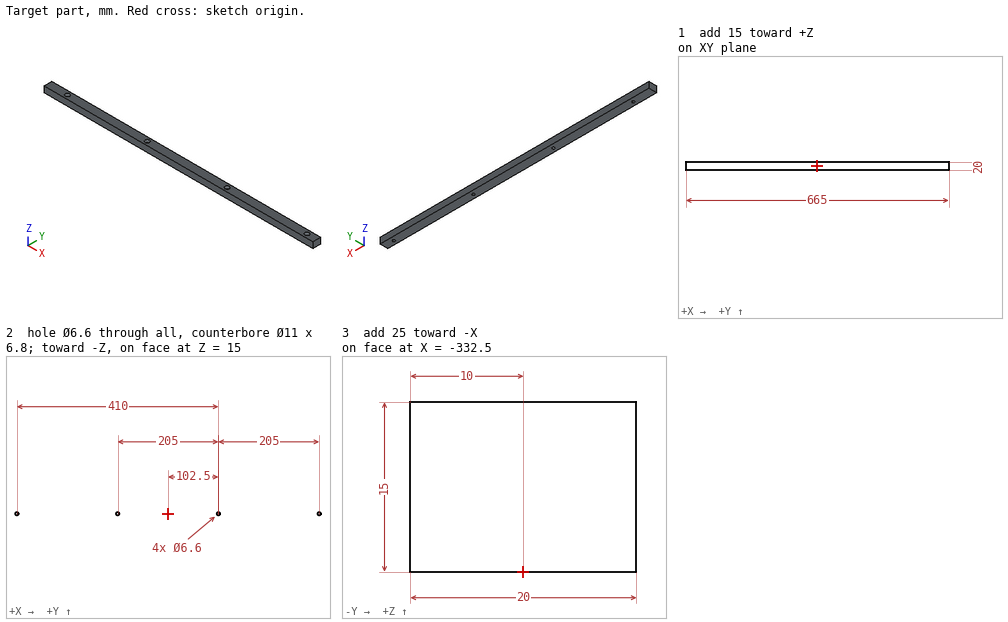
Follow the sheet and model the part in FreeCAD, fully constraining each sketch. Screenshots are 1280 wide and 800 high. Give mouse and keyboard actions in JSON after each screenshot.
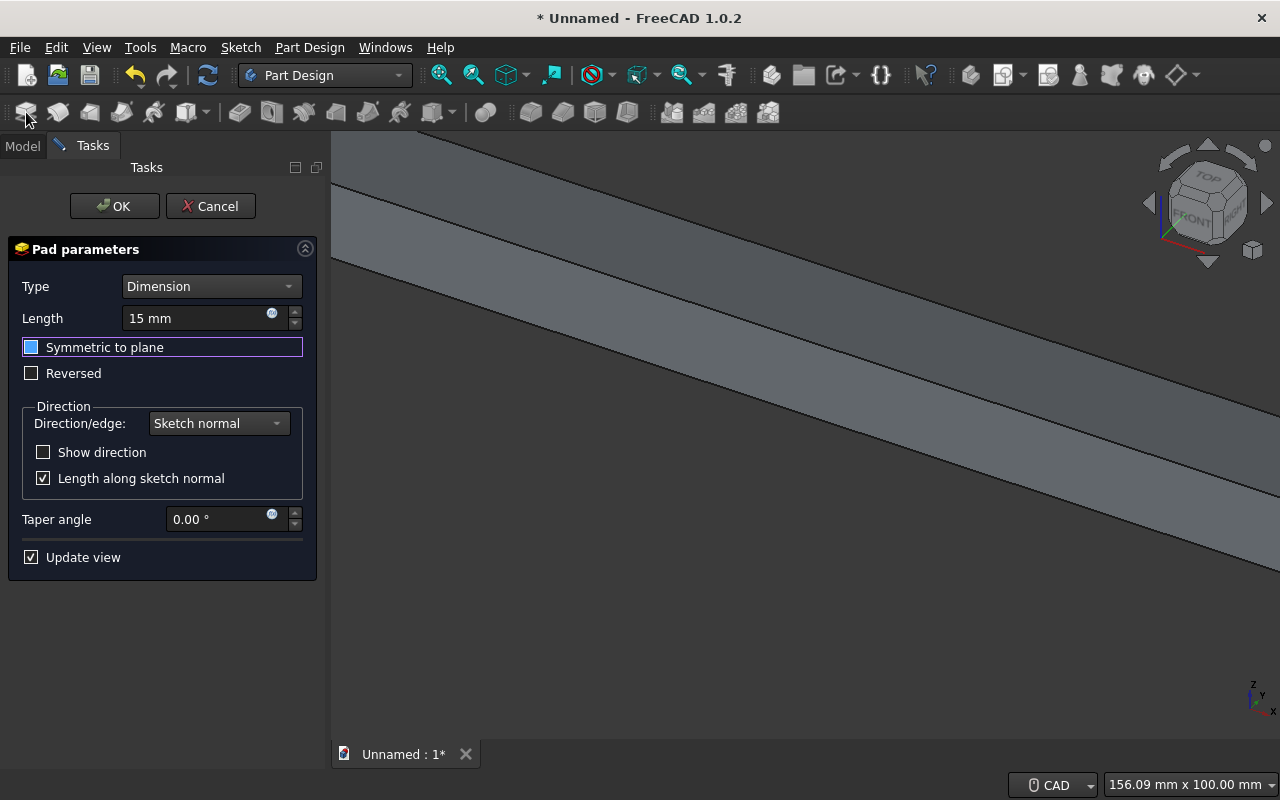
{"action": "left_click", "coordinate": [115, 206]}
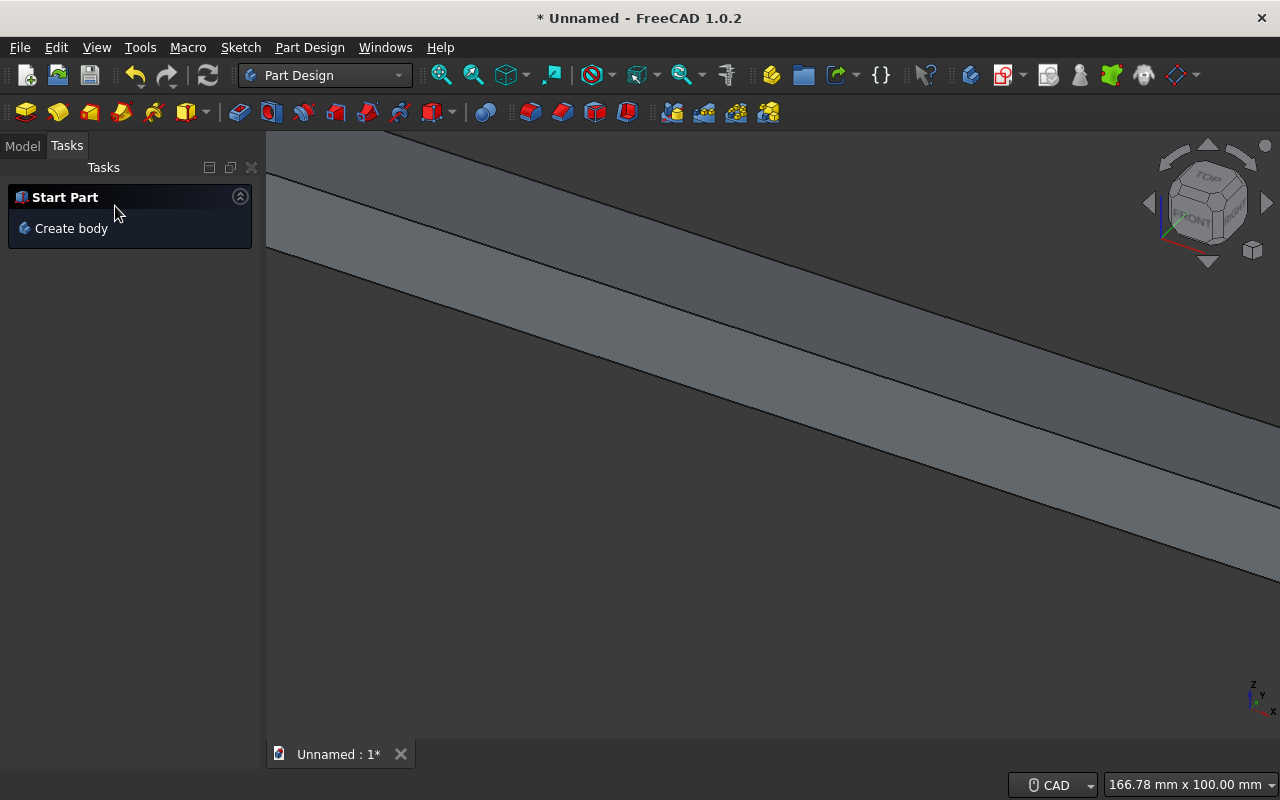
{"action": "key", "text": "v f"}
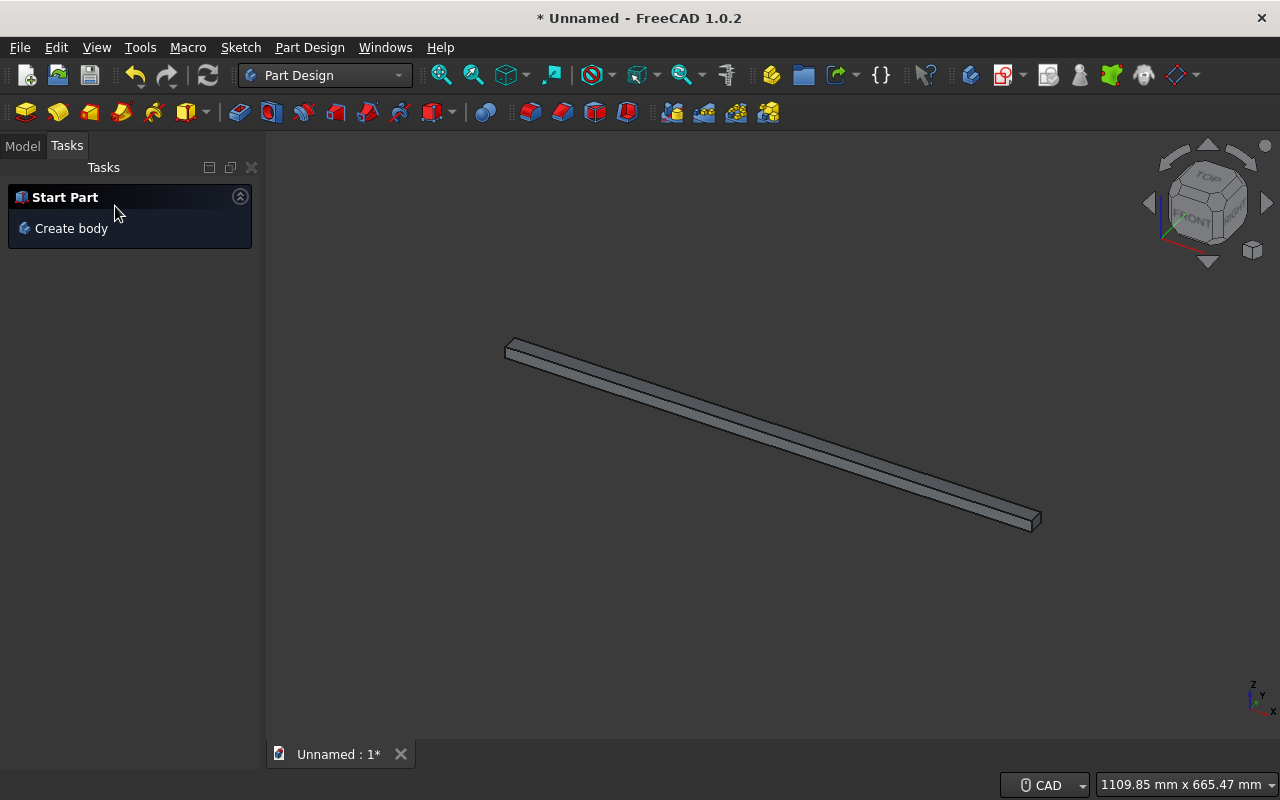
{"action": "key", "text": "0"}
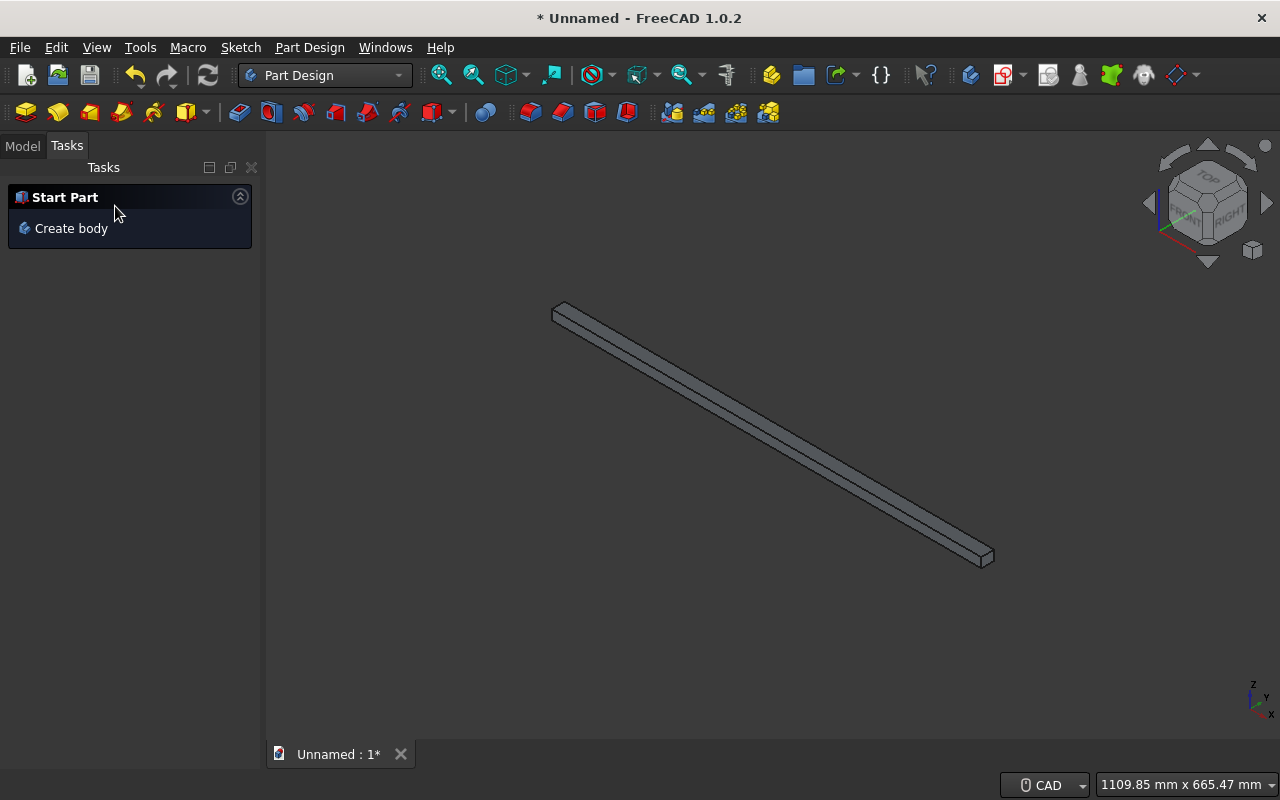
{"action": "key", "text": "v f"}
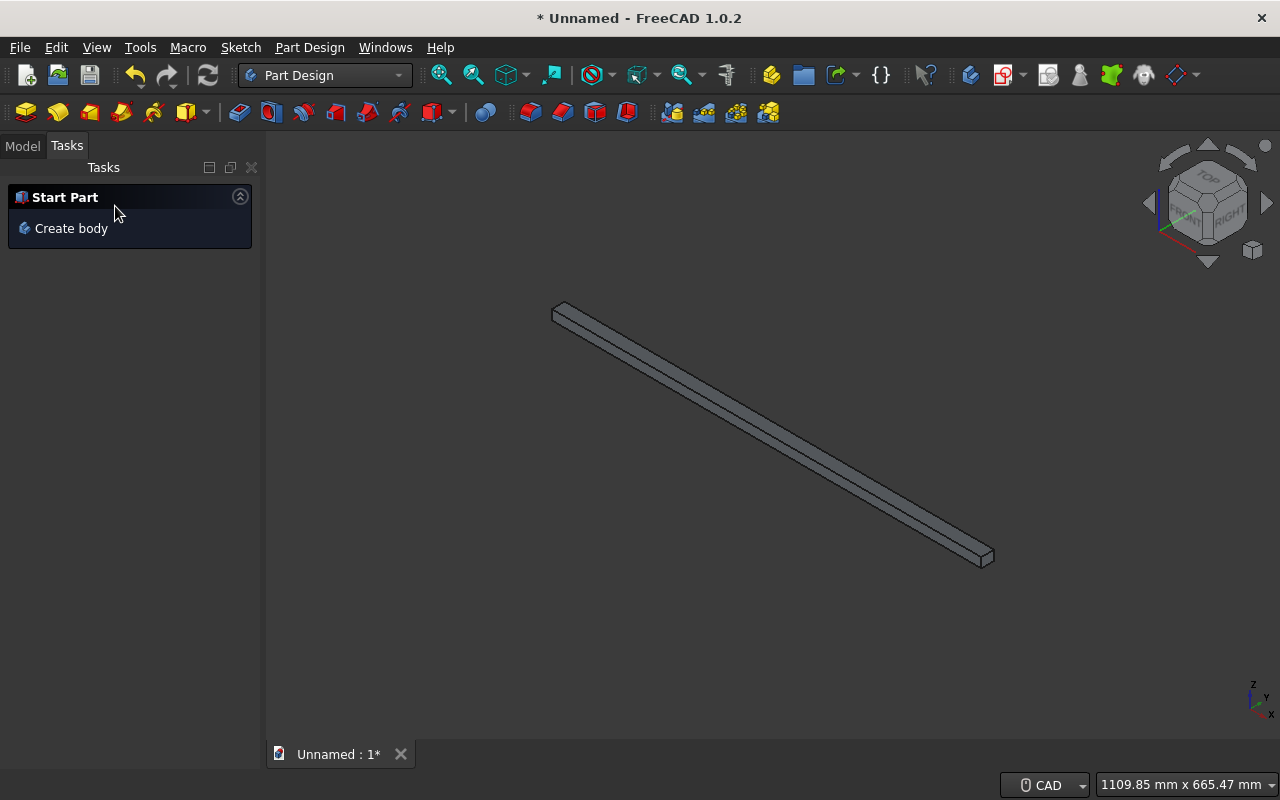
{"action": "key", "text": "2"}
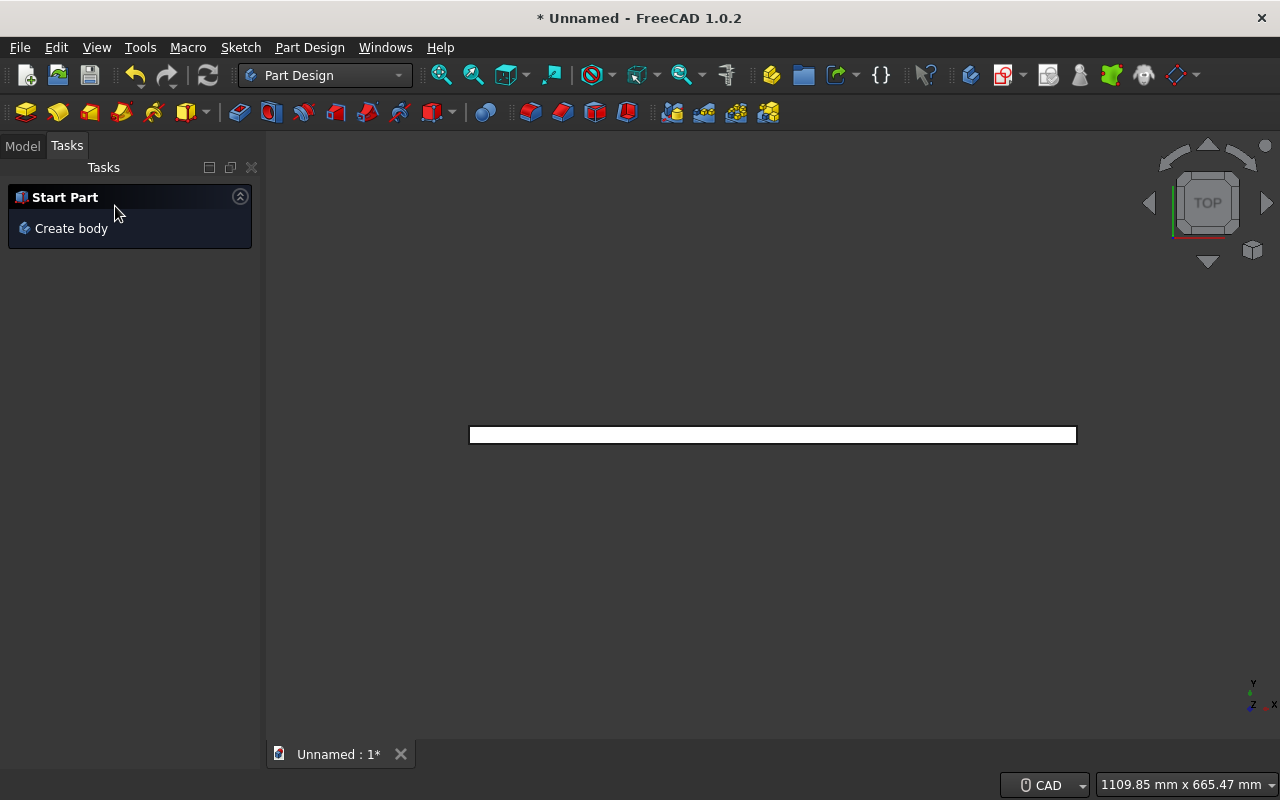
{"action": "left_click", "coordinate": [1033, 434]}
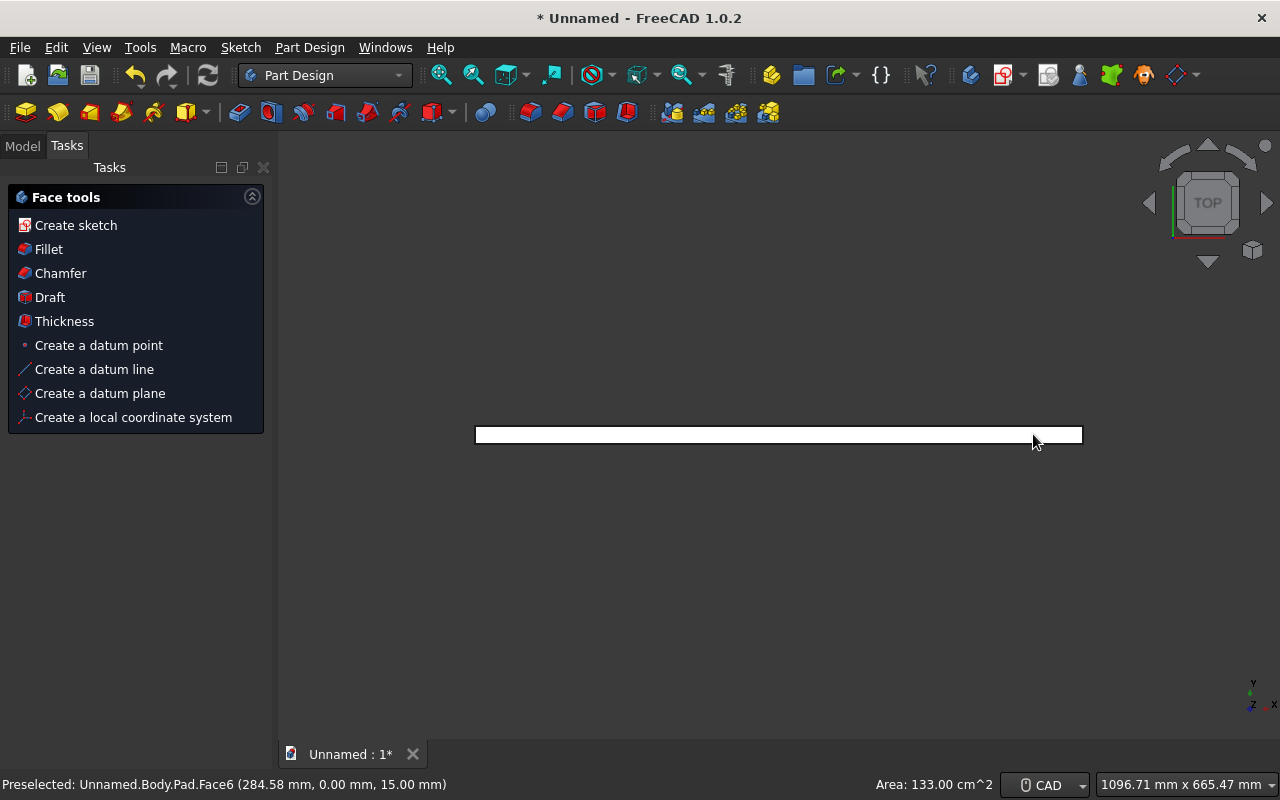
{"action": "left_click", "coordinate": [1004, 76]}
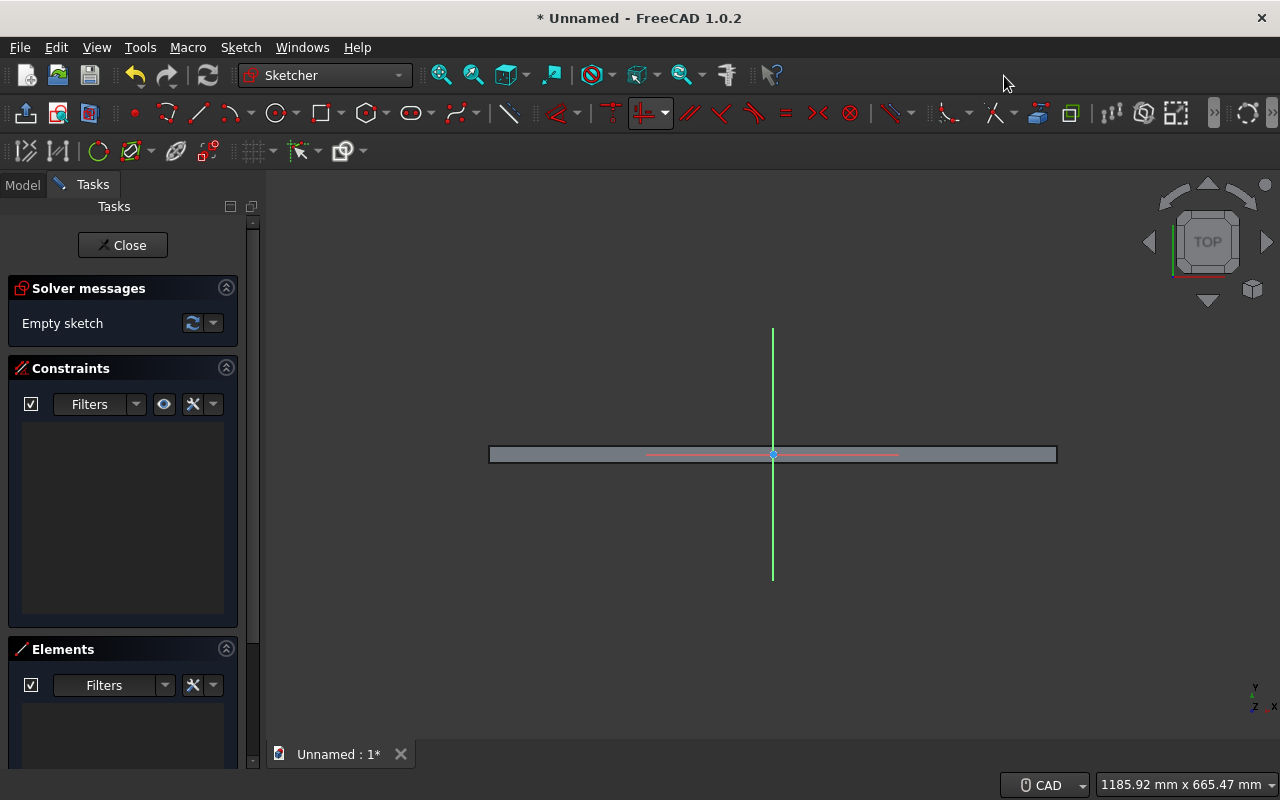
{"action": "left_click", "coordinate": [276, 114]}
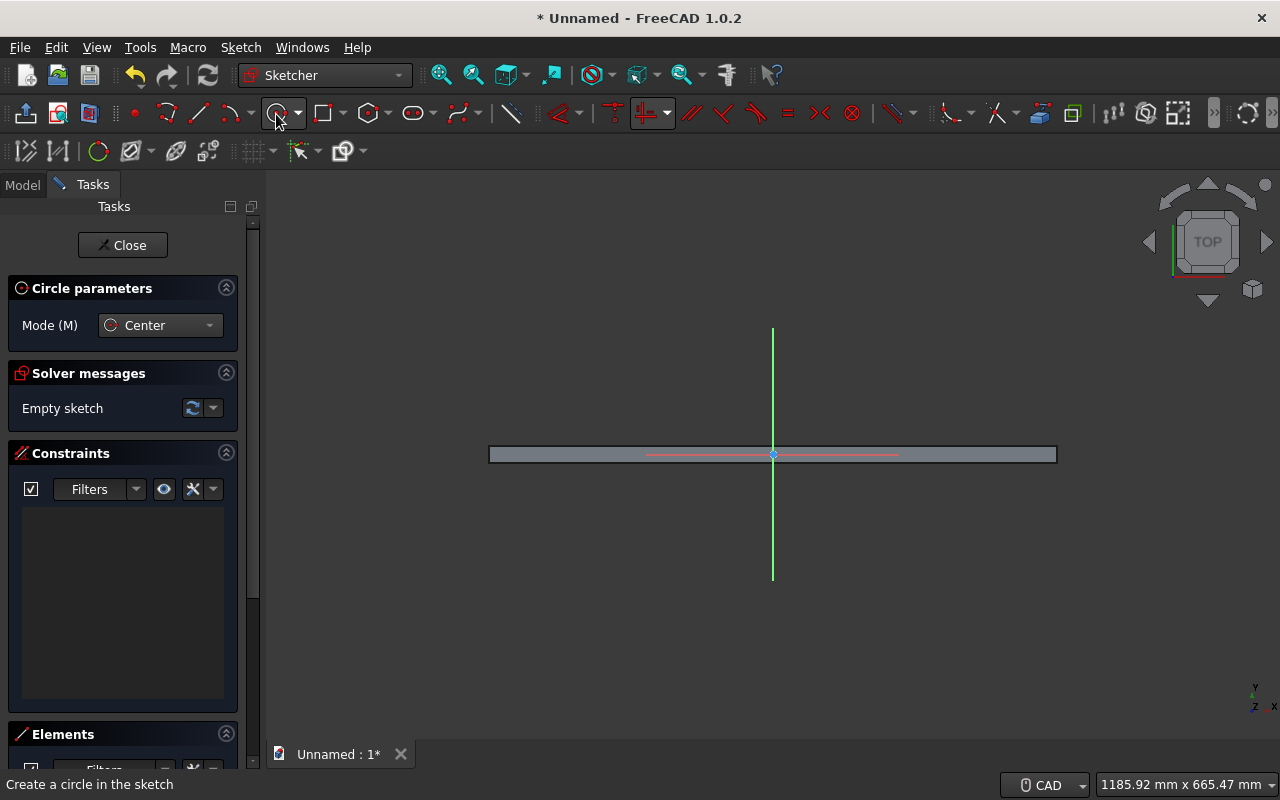
{"action": "scroll", "coordinate": [861, 454], "scroll_direction": "up", "scroll_amount": 11}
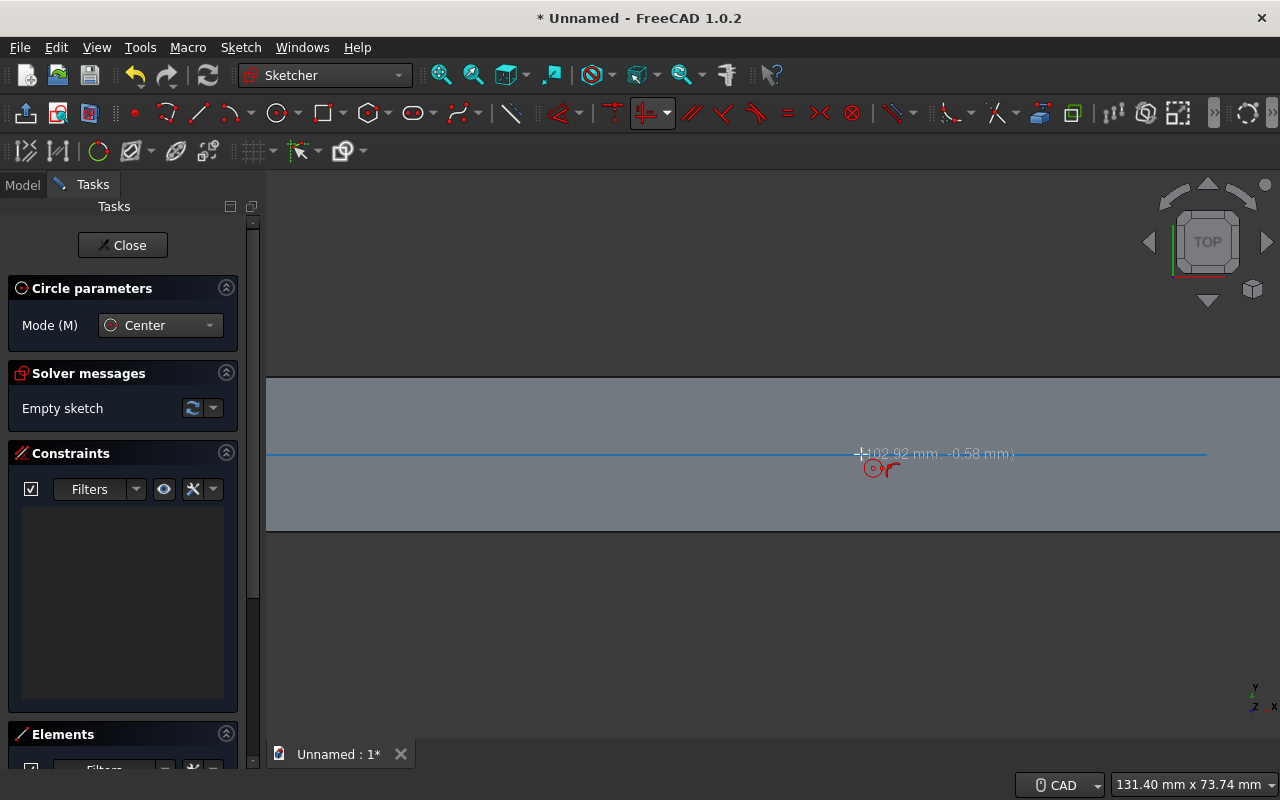
{"action": "scroll", "coordinate": [785, 454], "scroll_direction": "down", "scroll_amount": 11}